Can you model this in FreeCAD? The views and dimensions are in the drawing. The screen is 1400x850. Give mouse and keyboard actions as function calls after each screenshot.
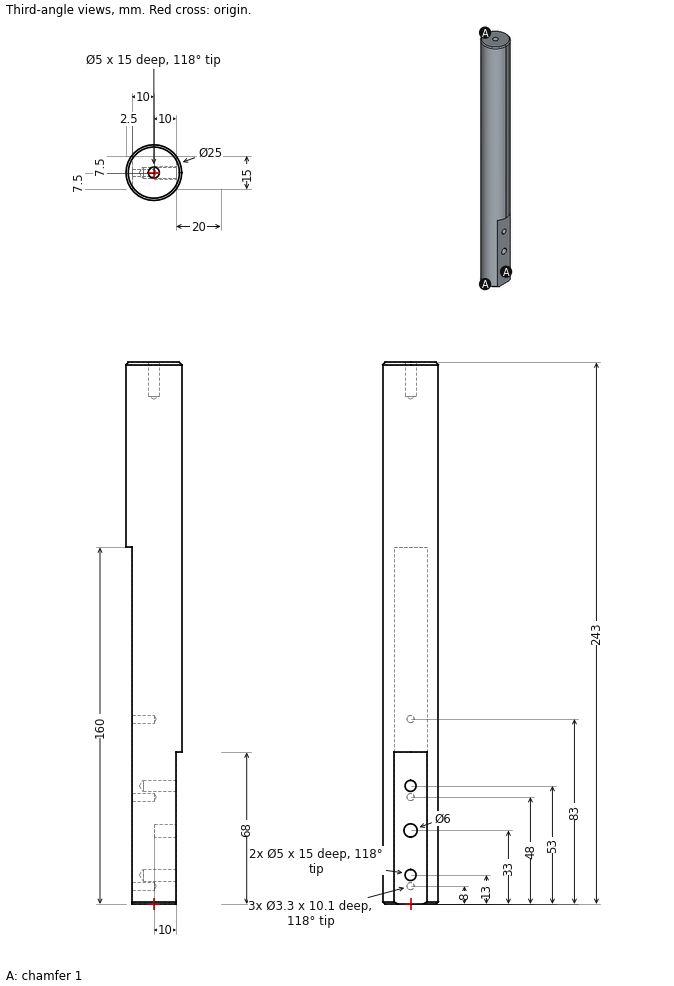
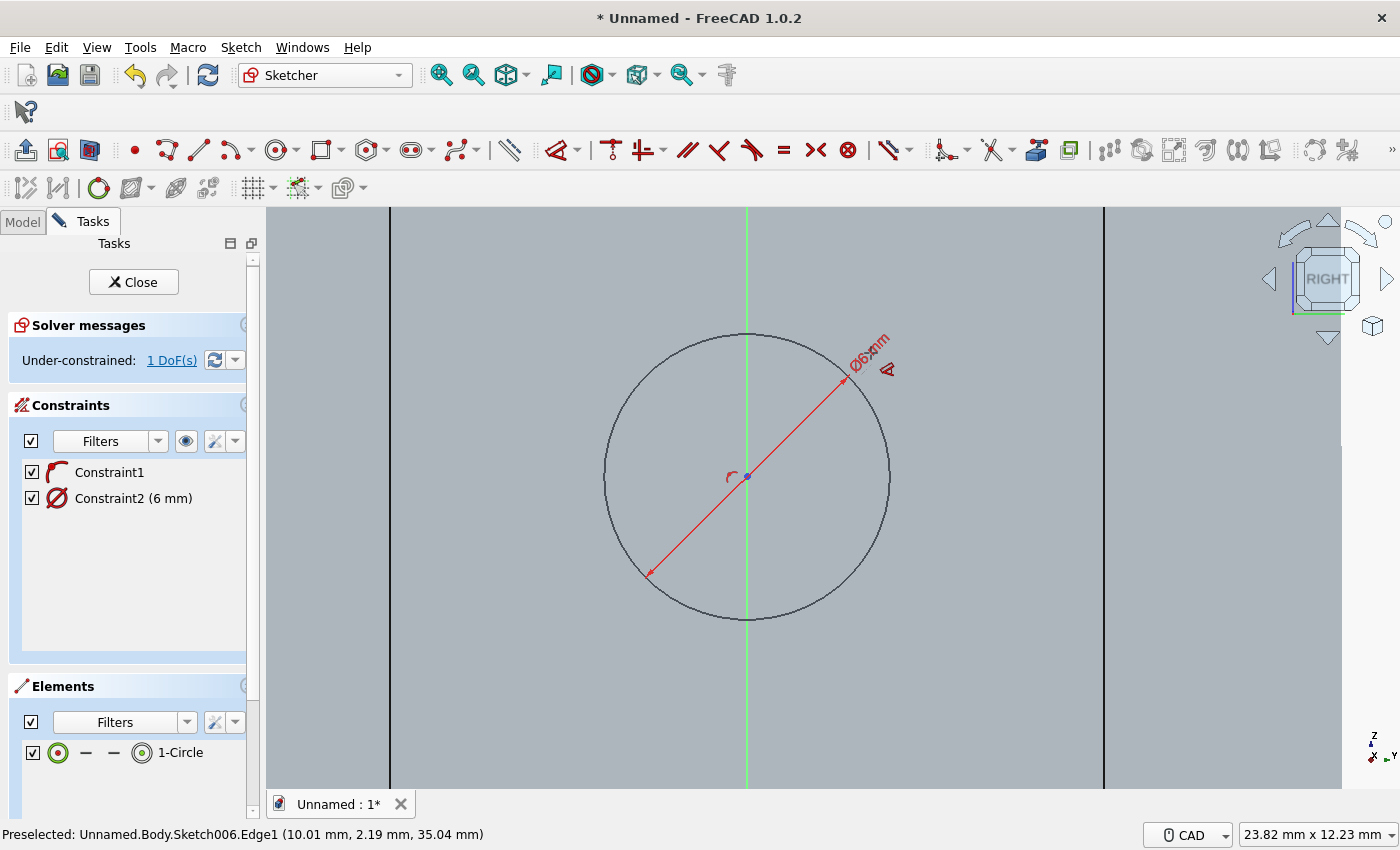
click(747, 477)
click(781, 554)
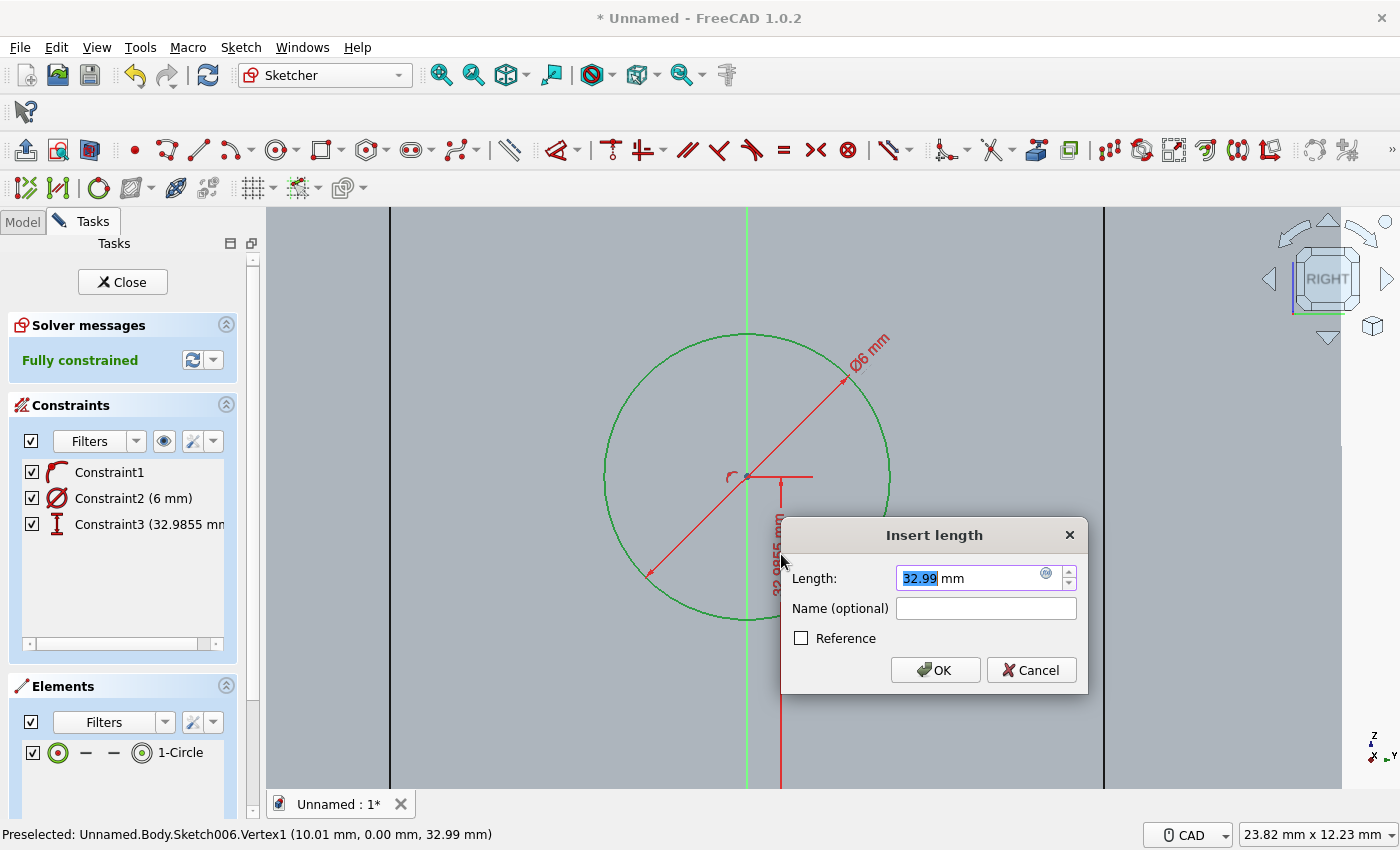
text(33)
key(Return)
key(Escape)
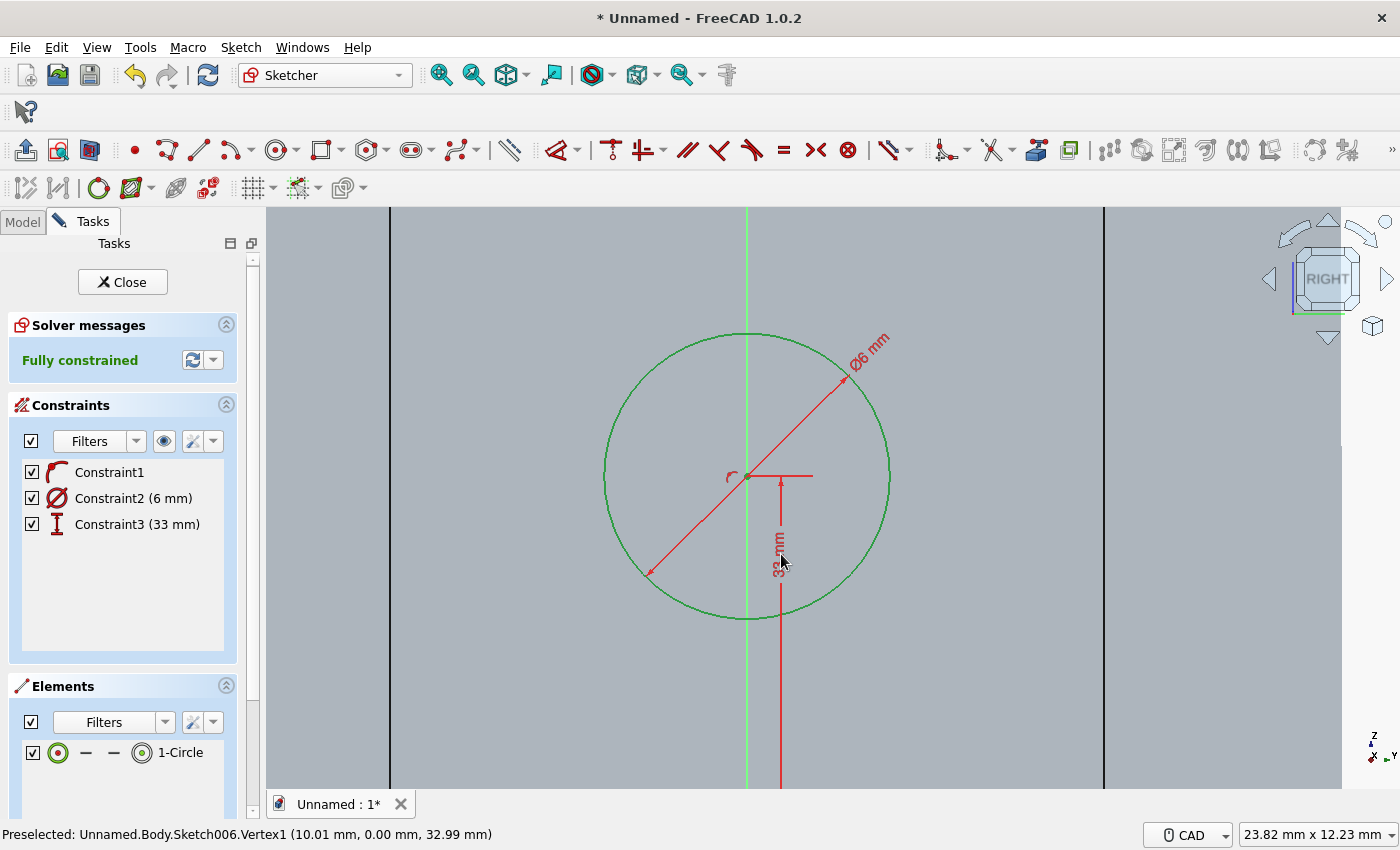
click(123, 282)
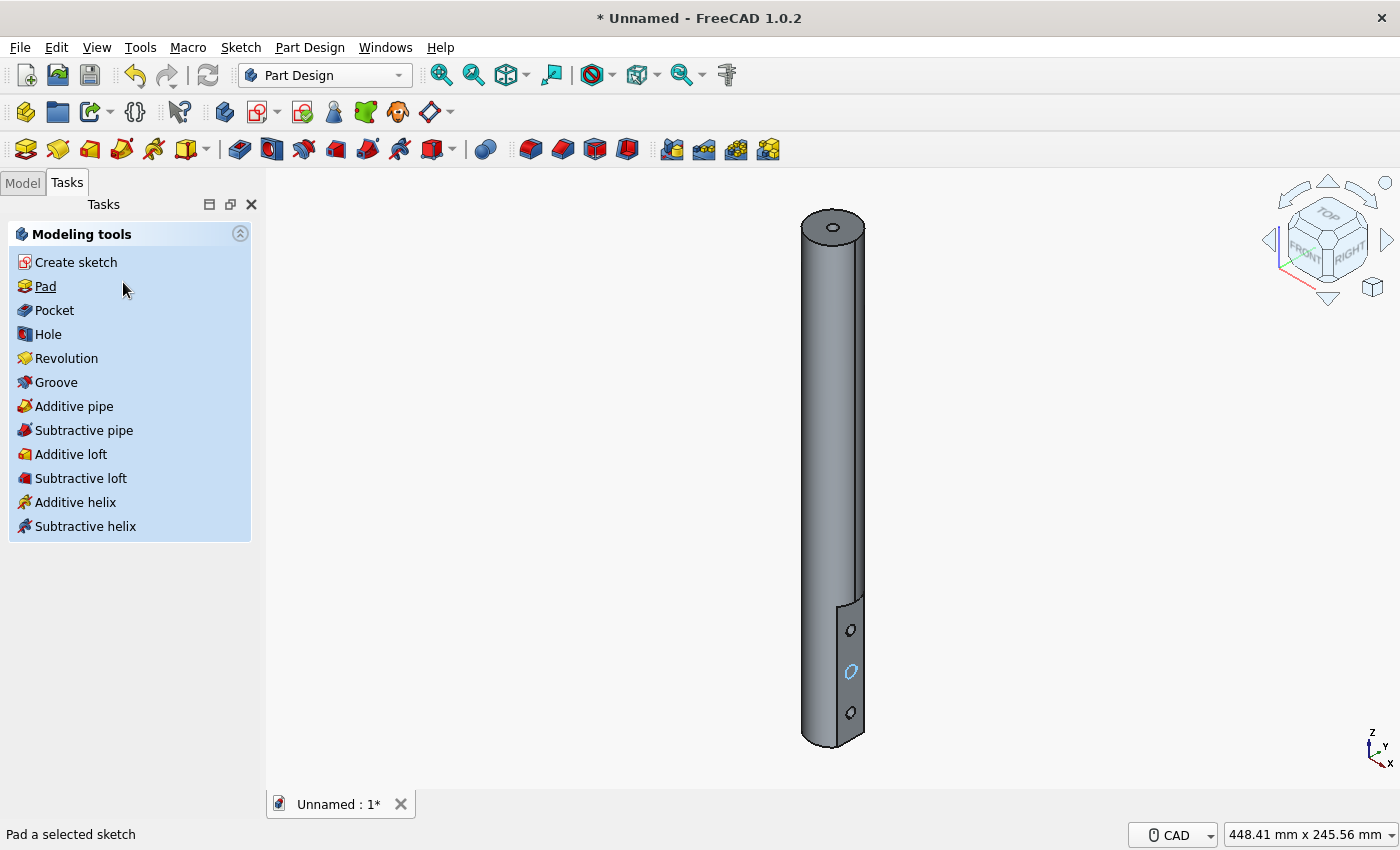
click(240, 150)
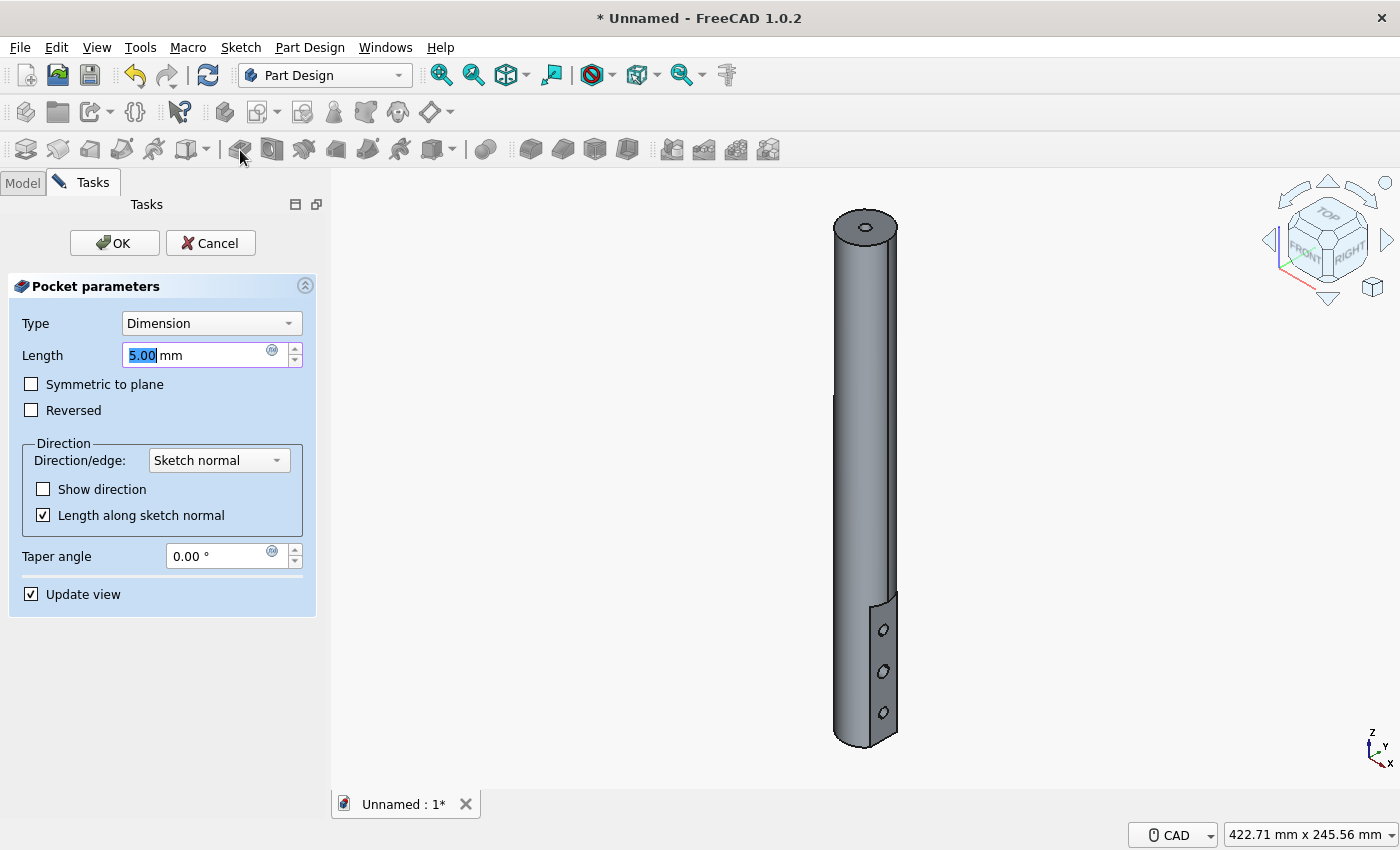
text(10)
key(Tab)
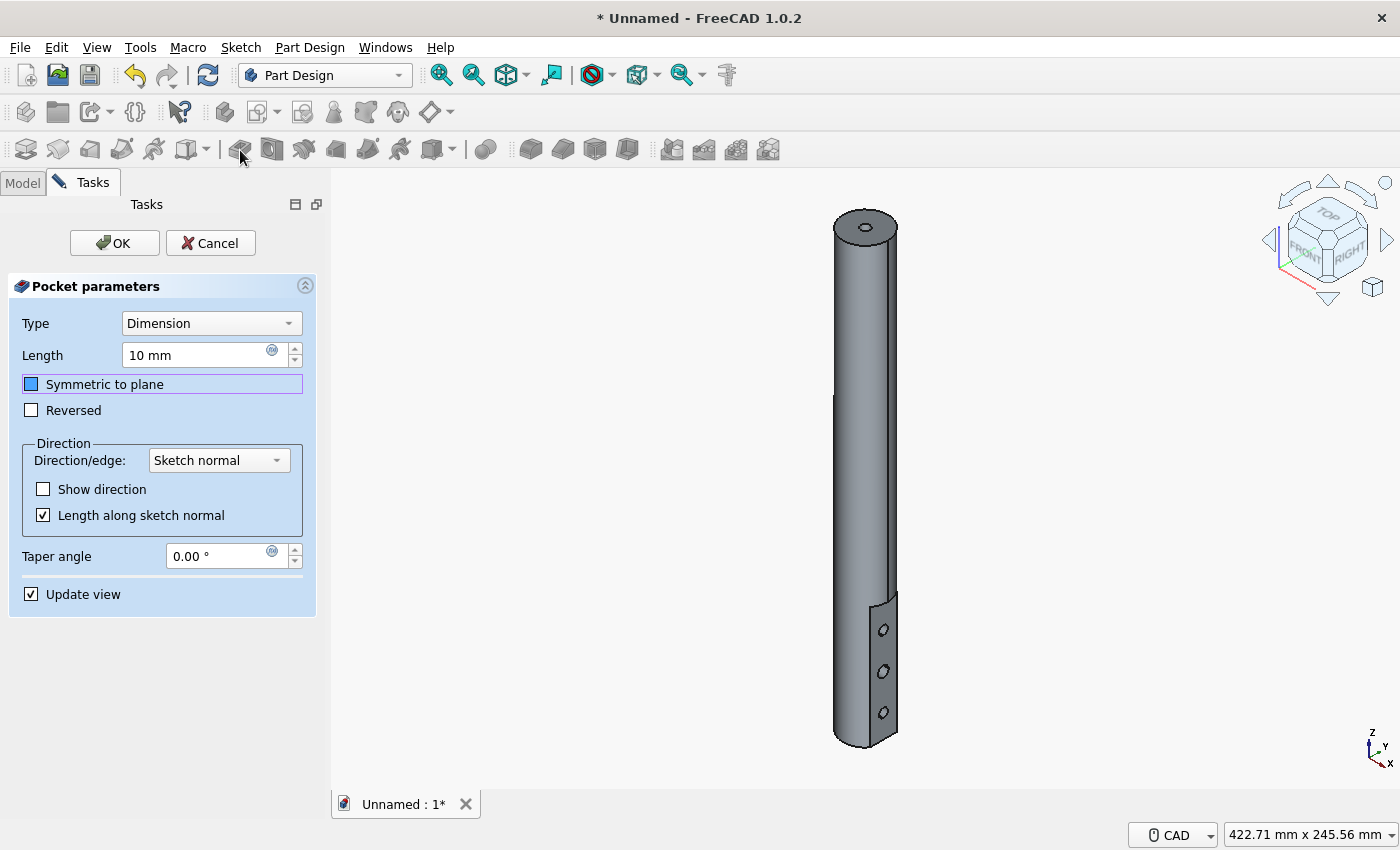
click(115, 243)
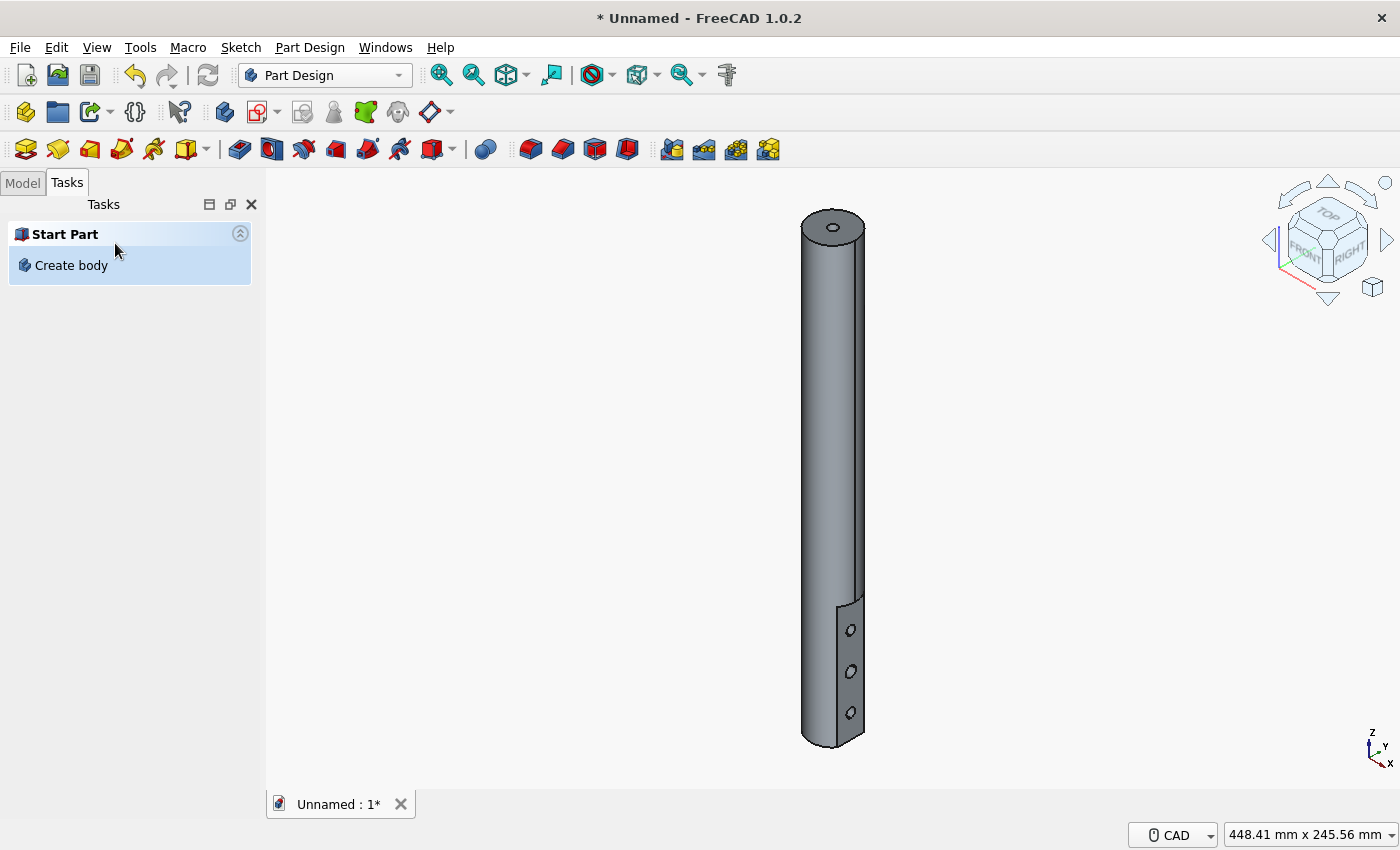
click(807, 739)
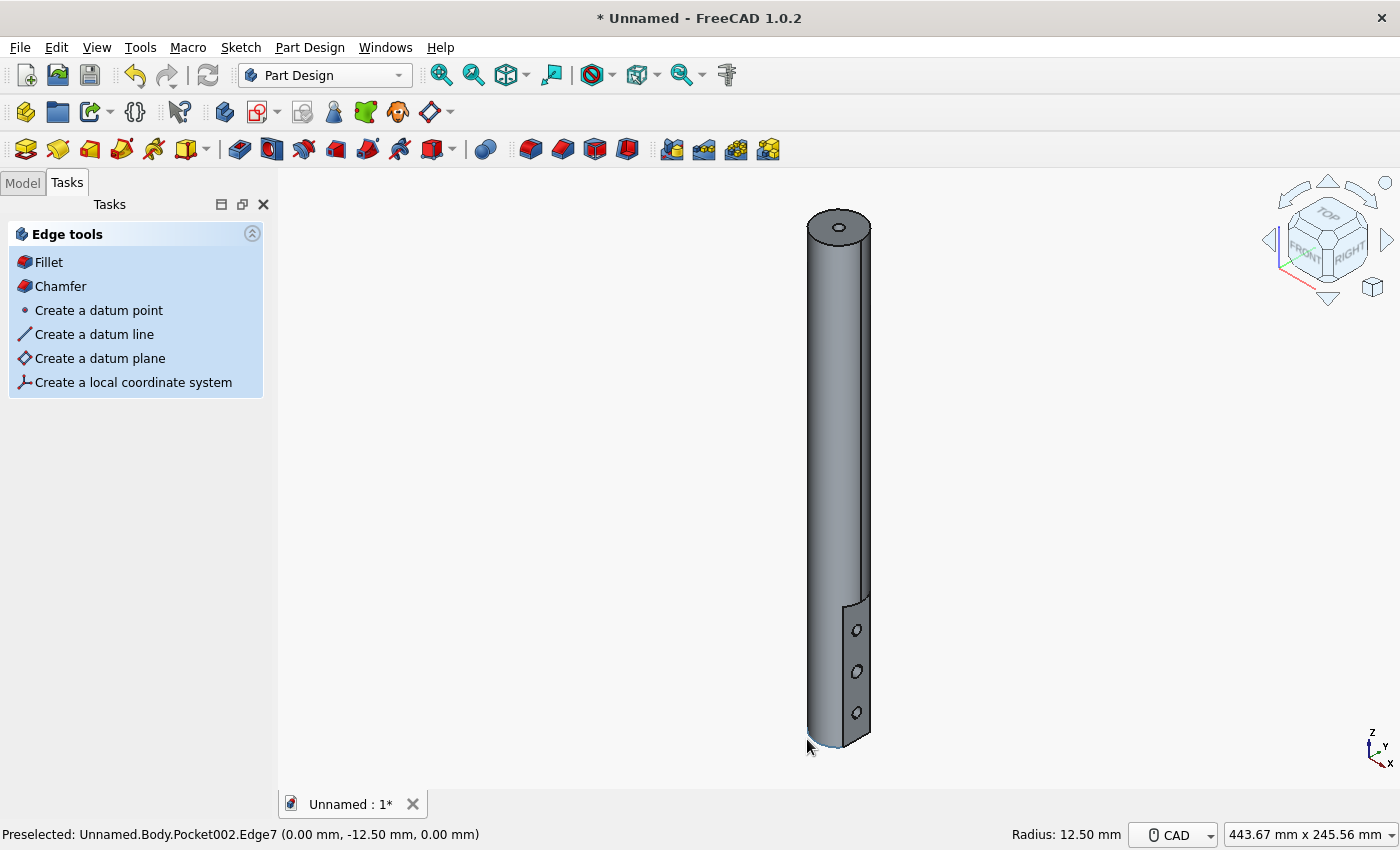
click(808, 224, ctrl)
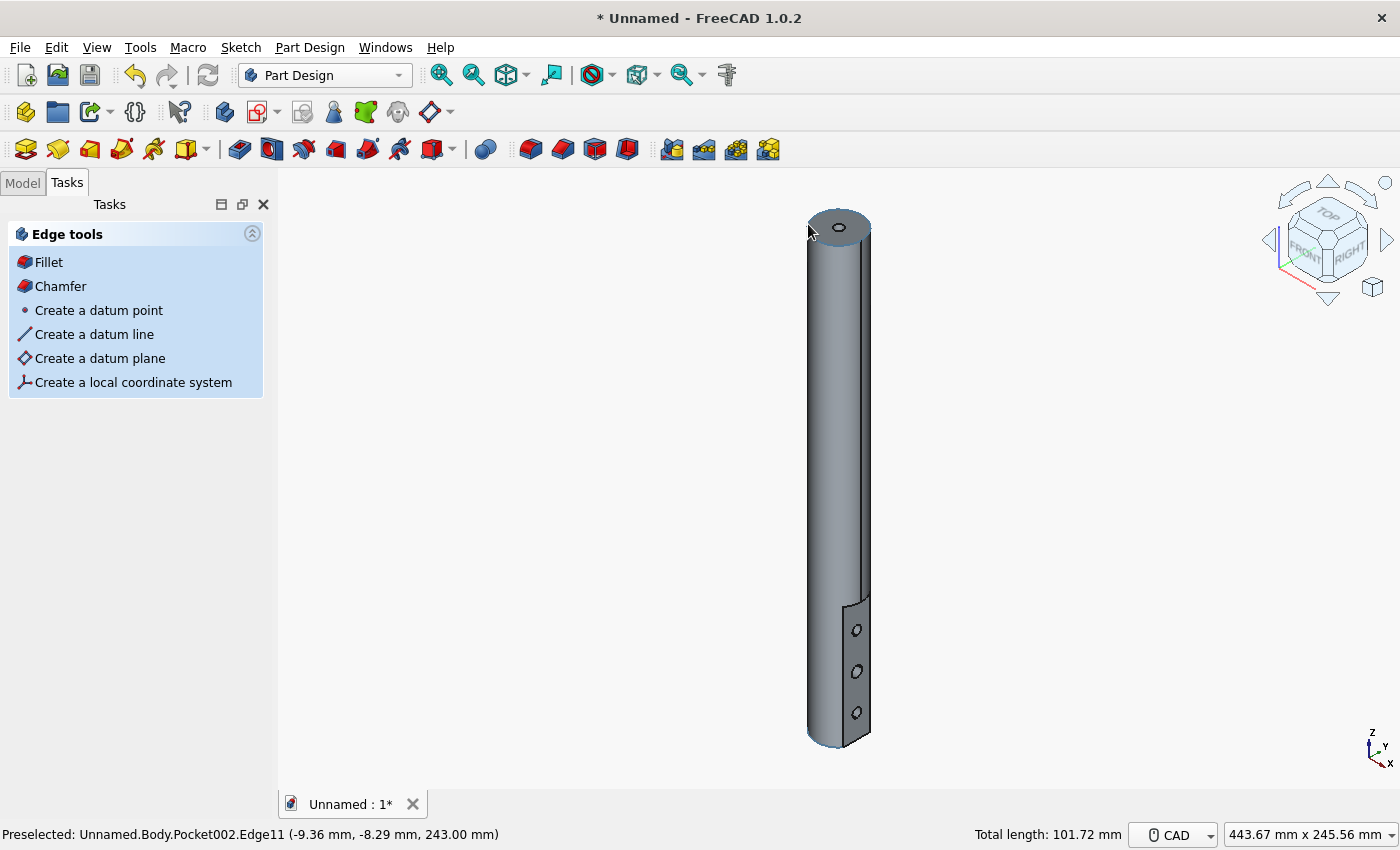
key(2)